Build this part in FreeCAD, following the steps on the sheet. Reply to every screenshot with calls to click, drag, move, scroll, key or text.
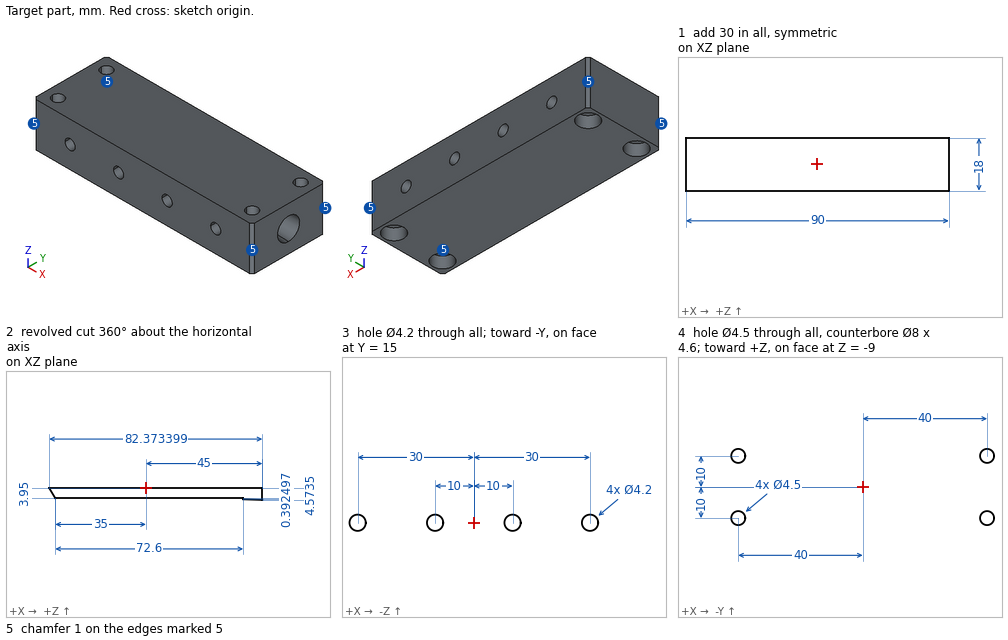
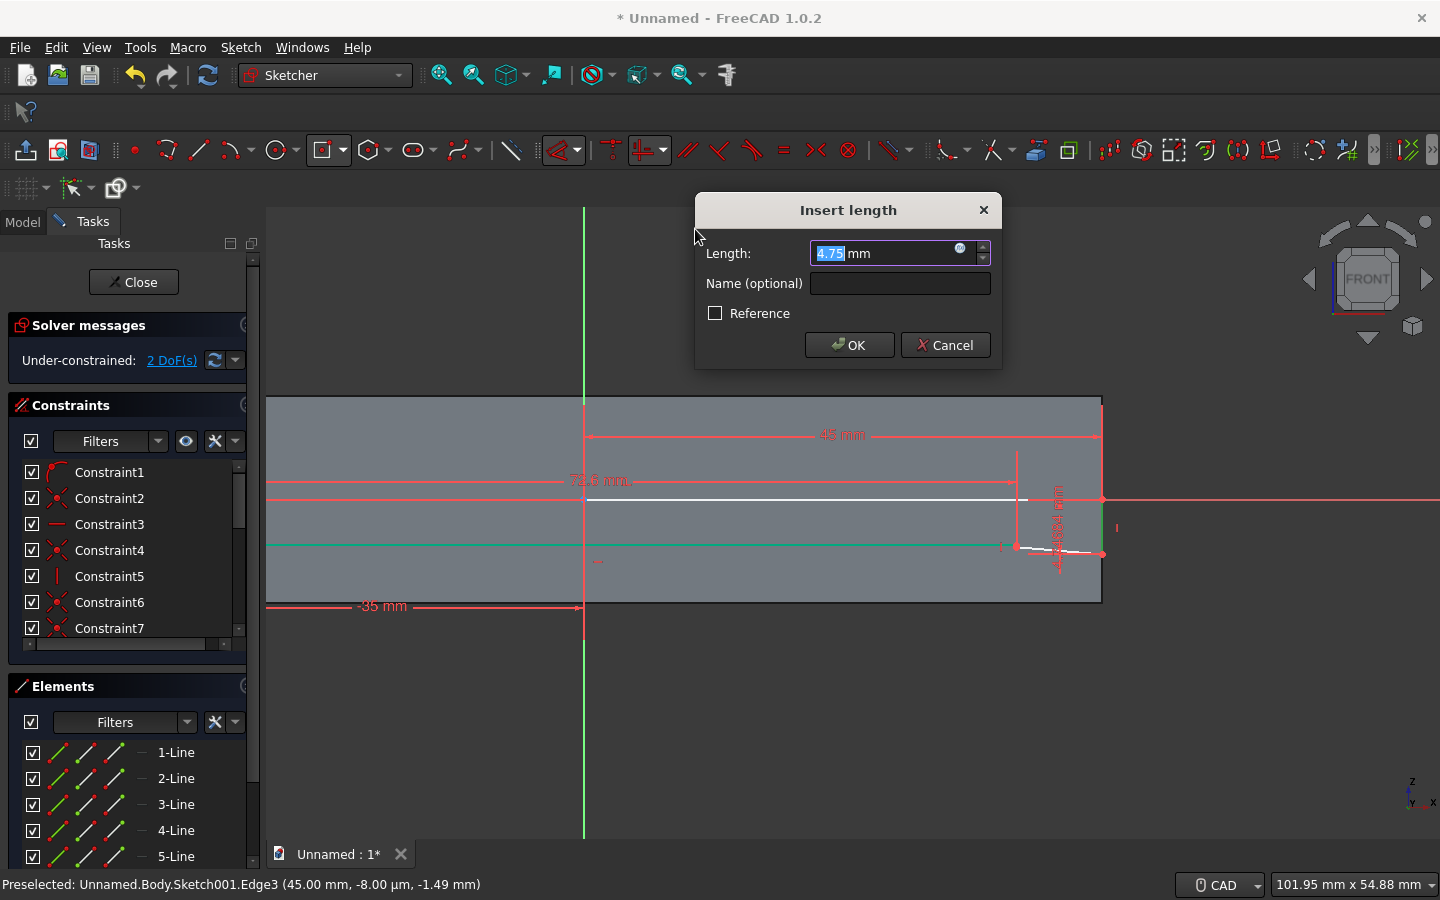
text(4.5735)
key(Return)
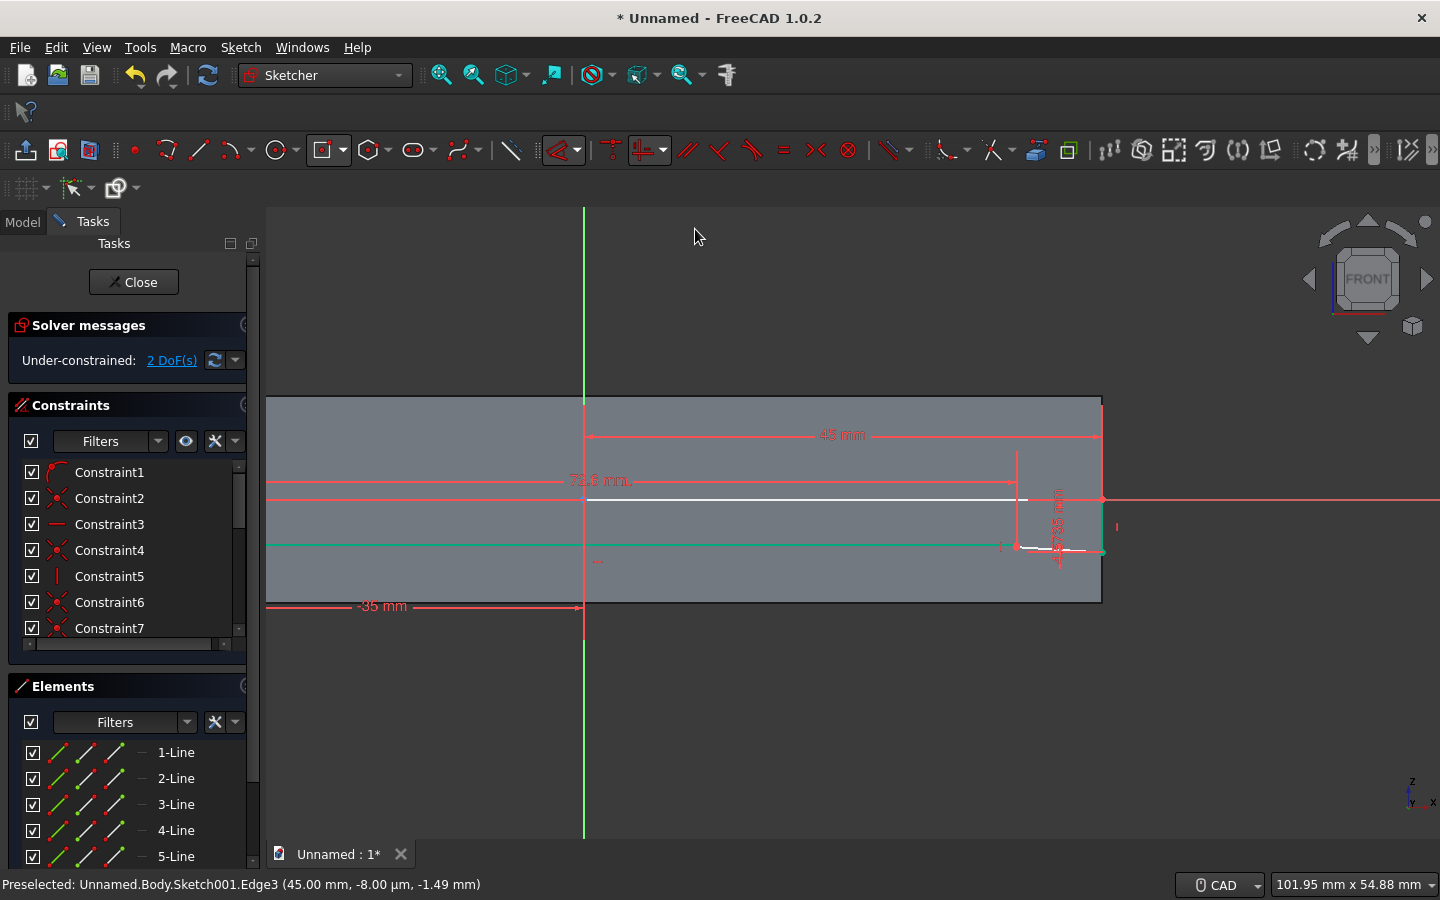
scroll(1017, 546, up, 11)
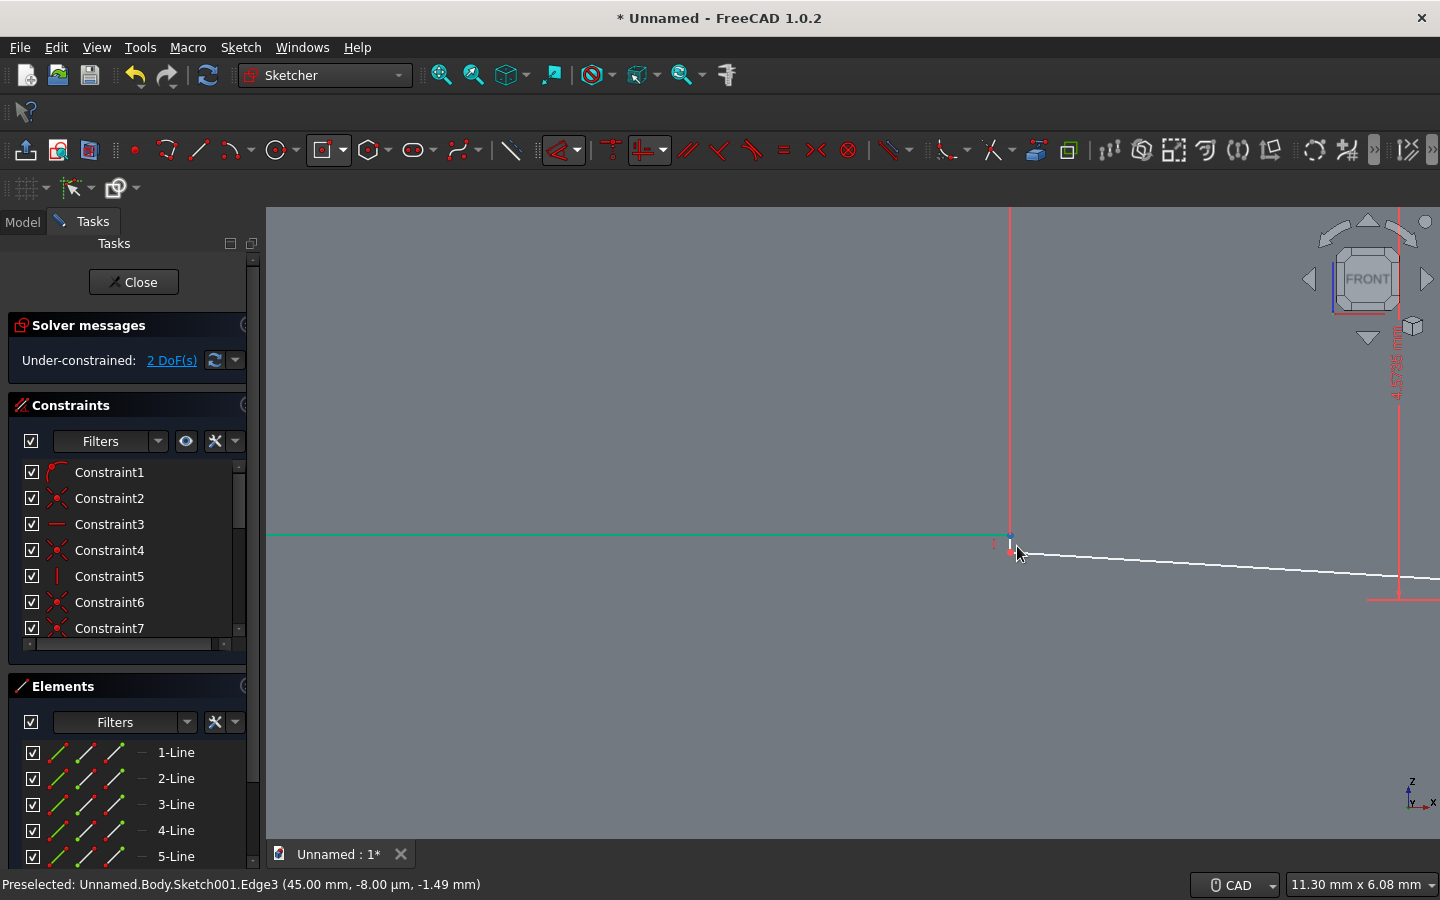
click(1010, 544)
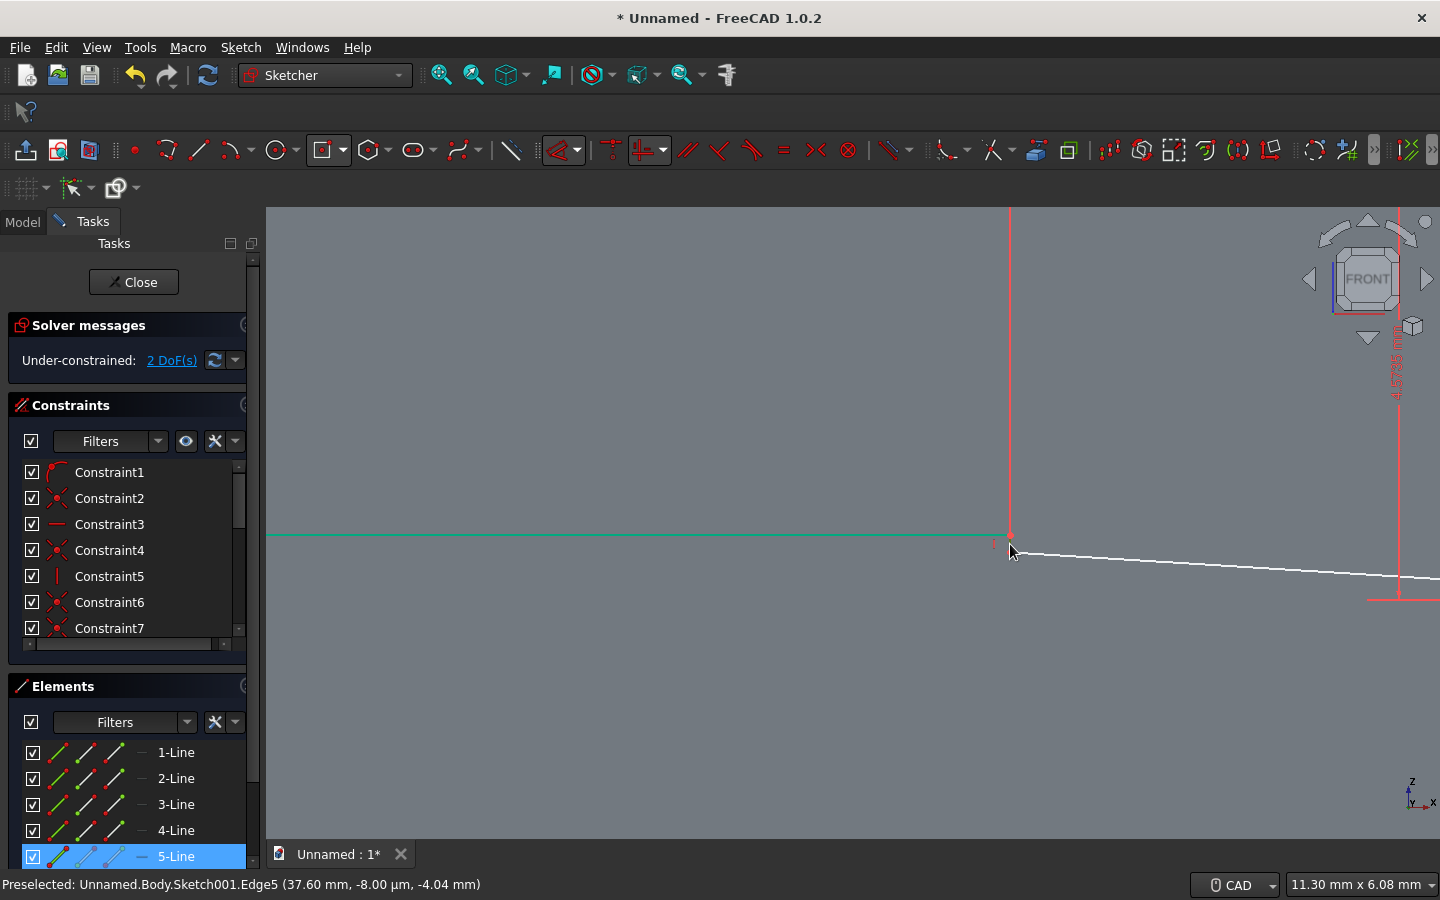
key(i)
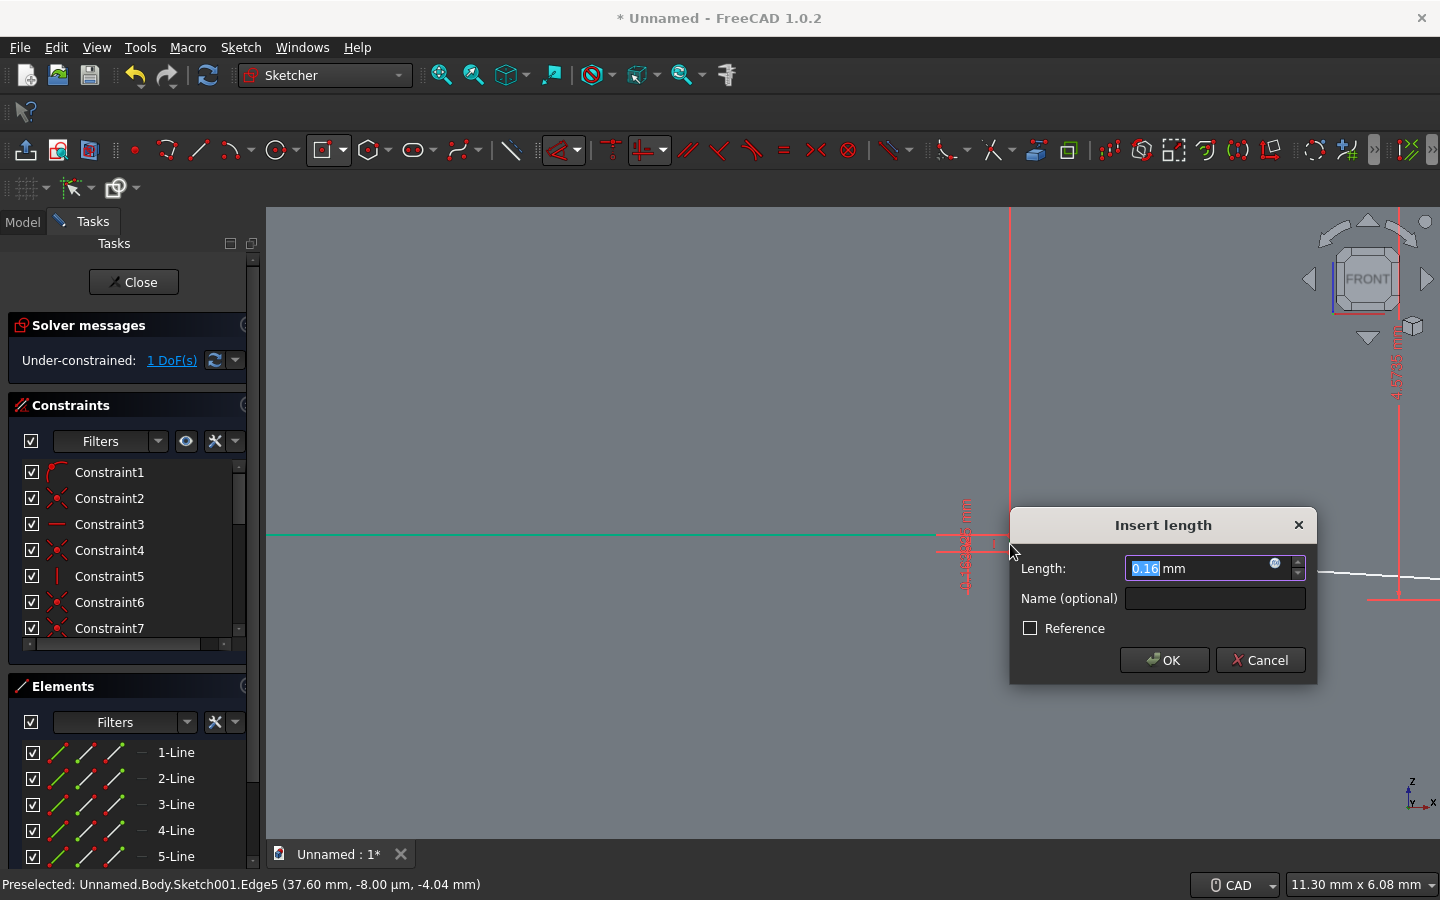
text(0.392497)
key(Return)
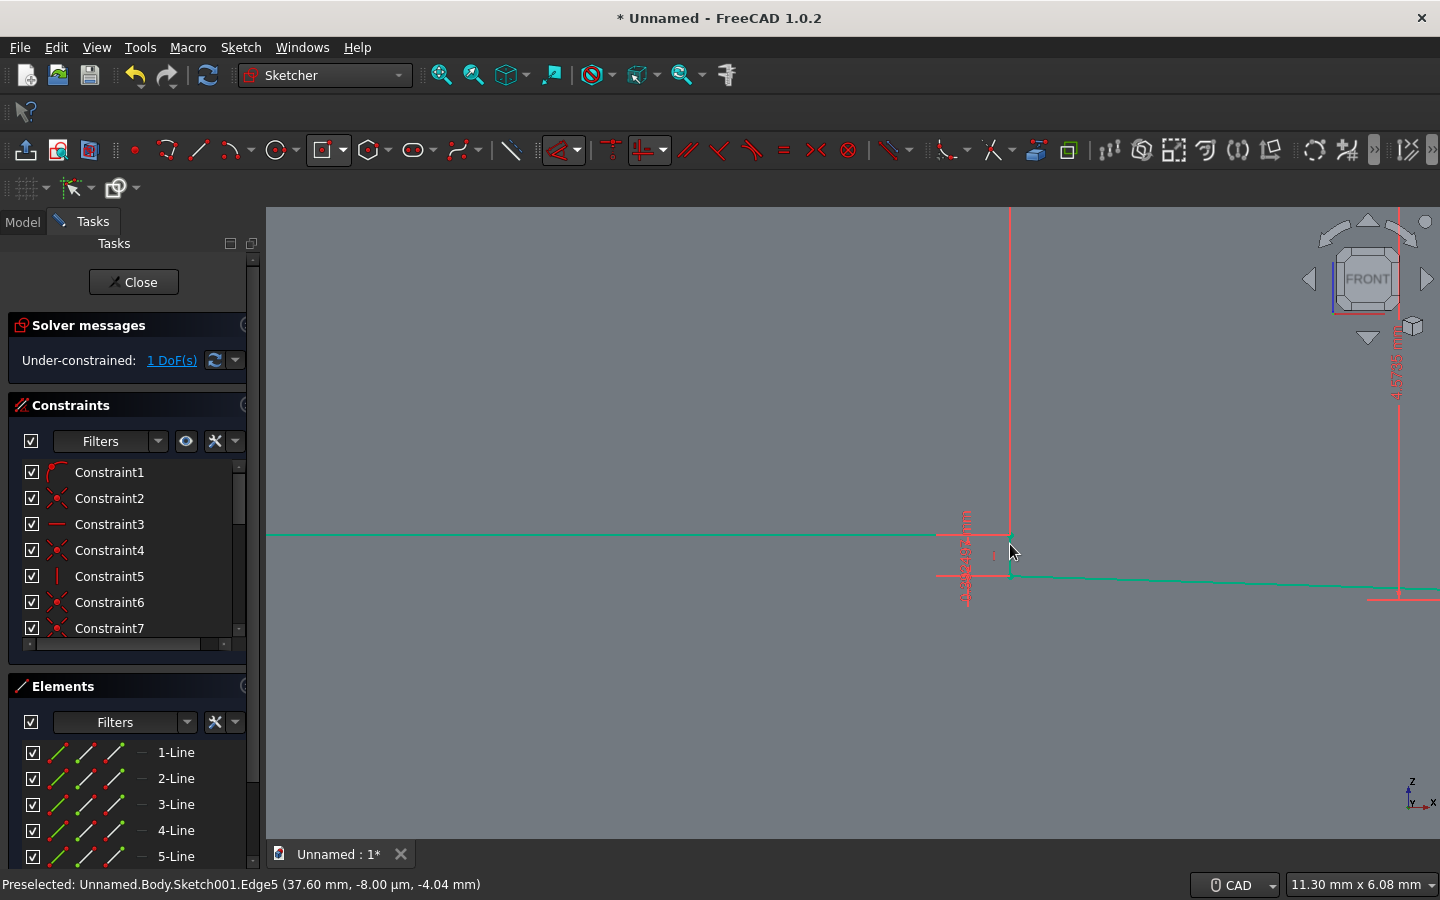
scroll(1048, 536, down, 13)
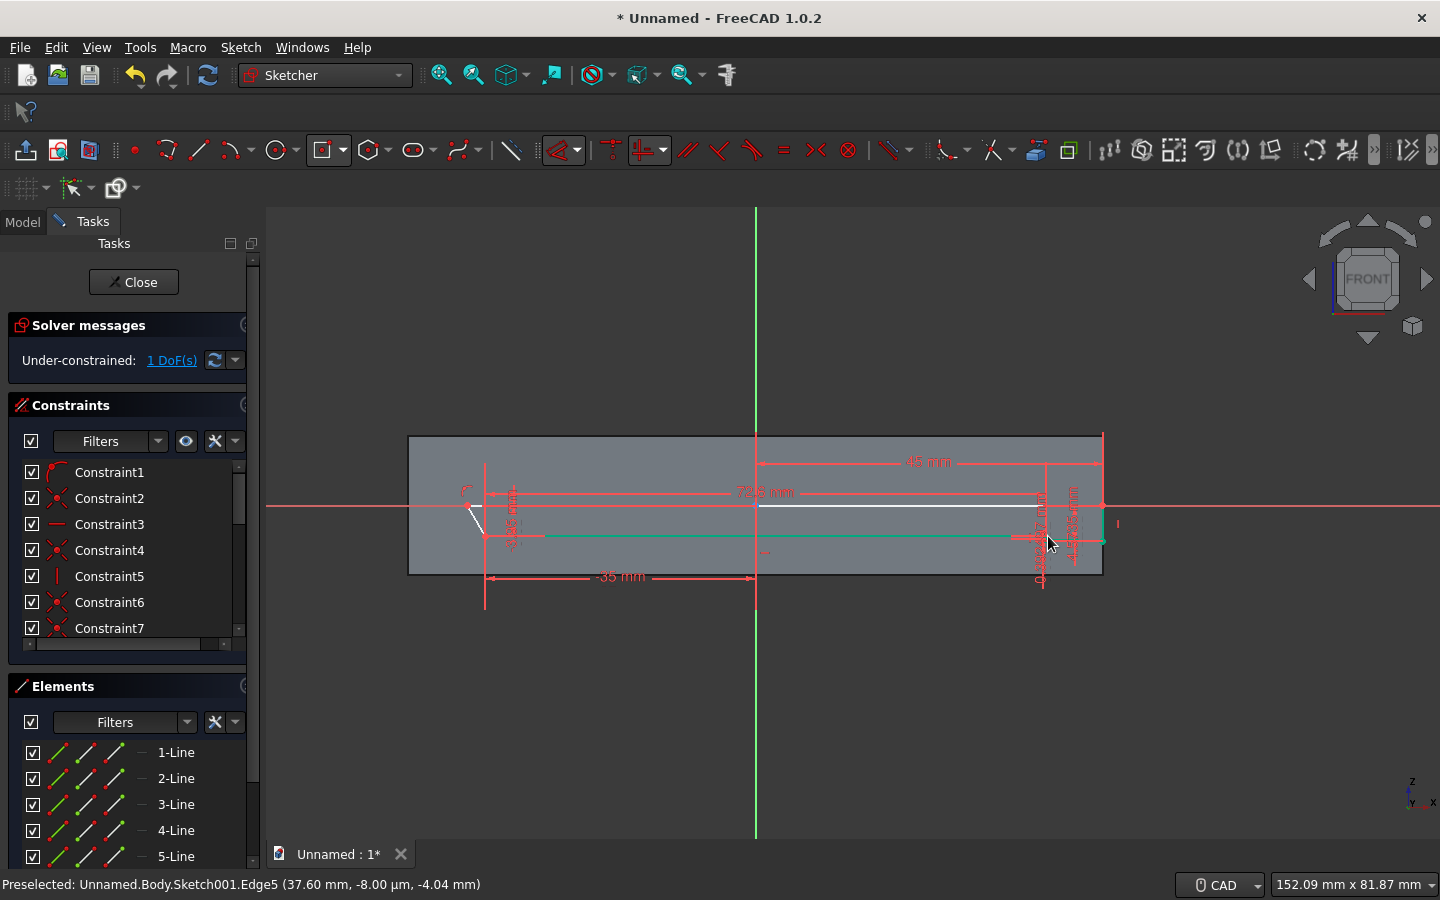
click(658, 506)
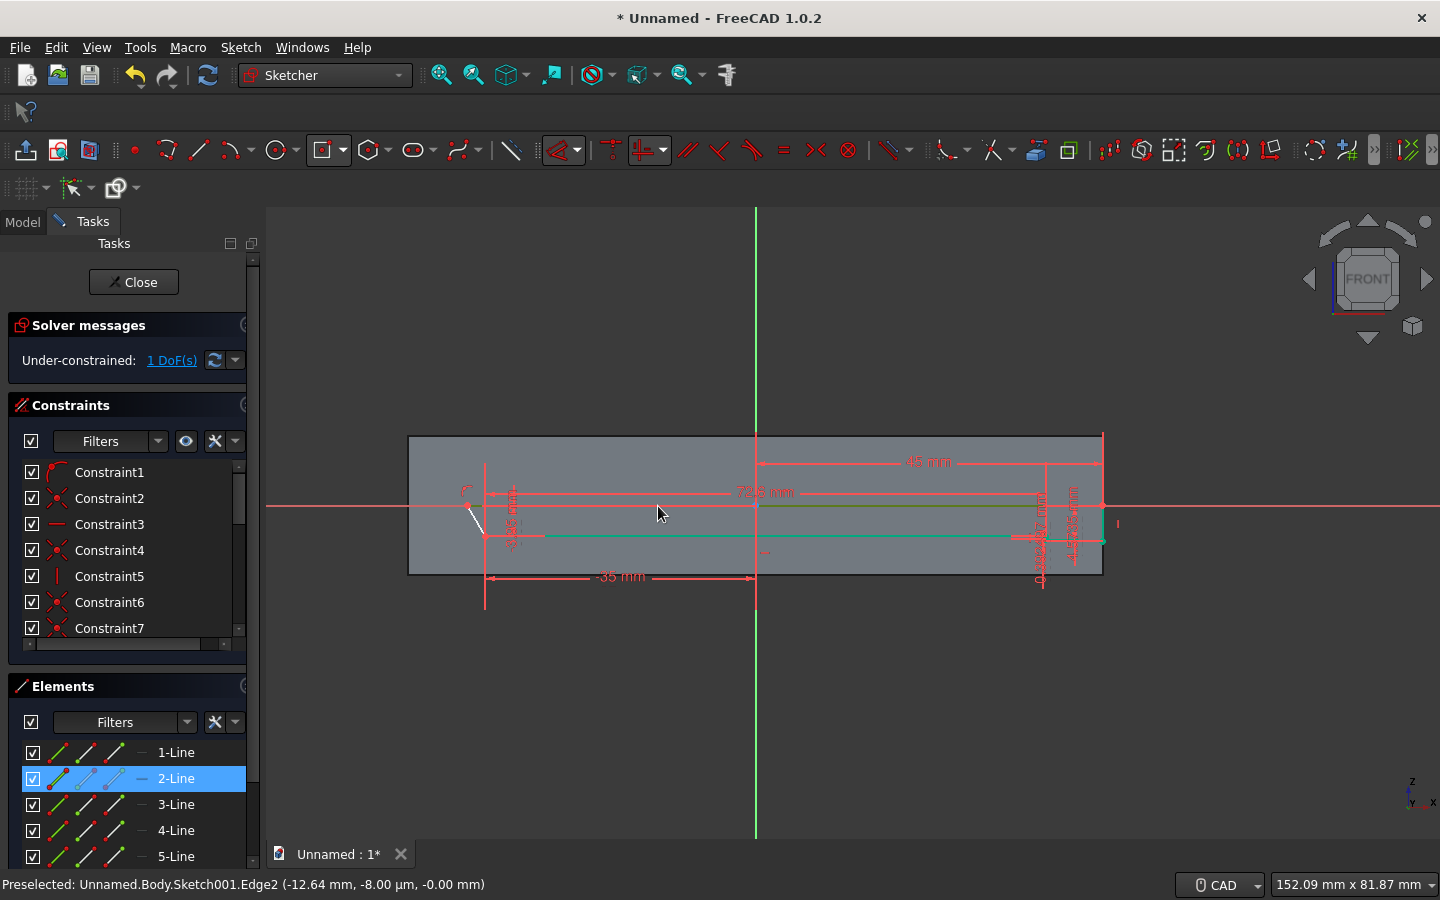
key(l)